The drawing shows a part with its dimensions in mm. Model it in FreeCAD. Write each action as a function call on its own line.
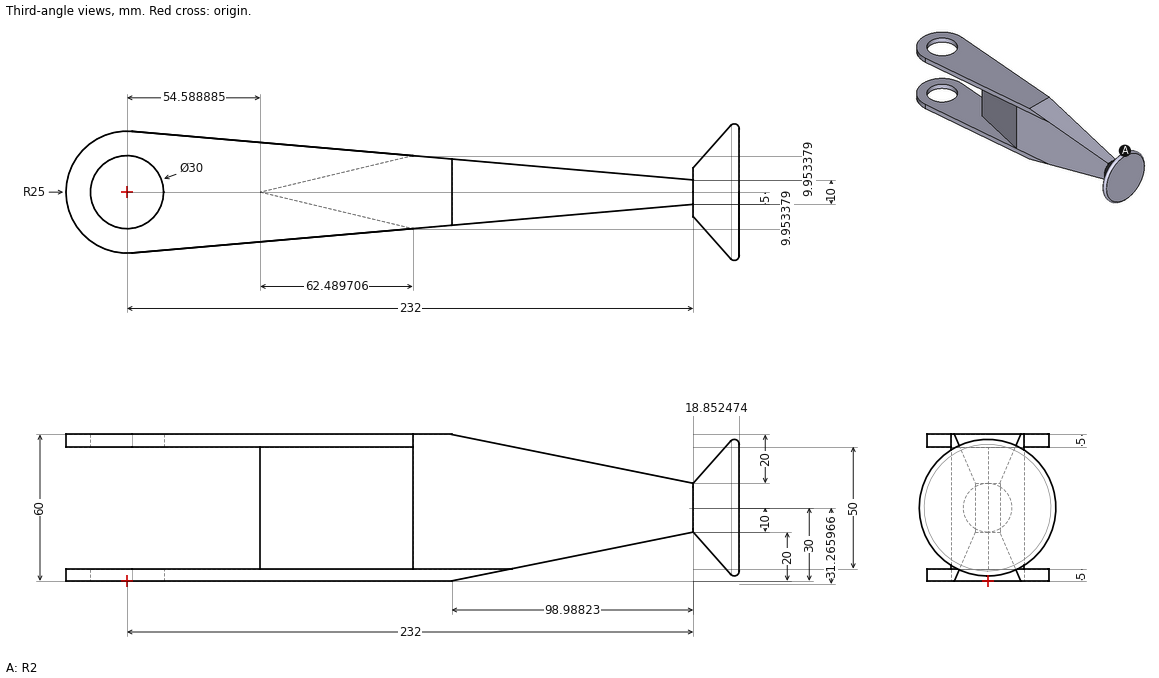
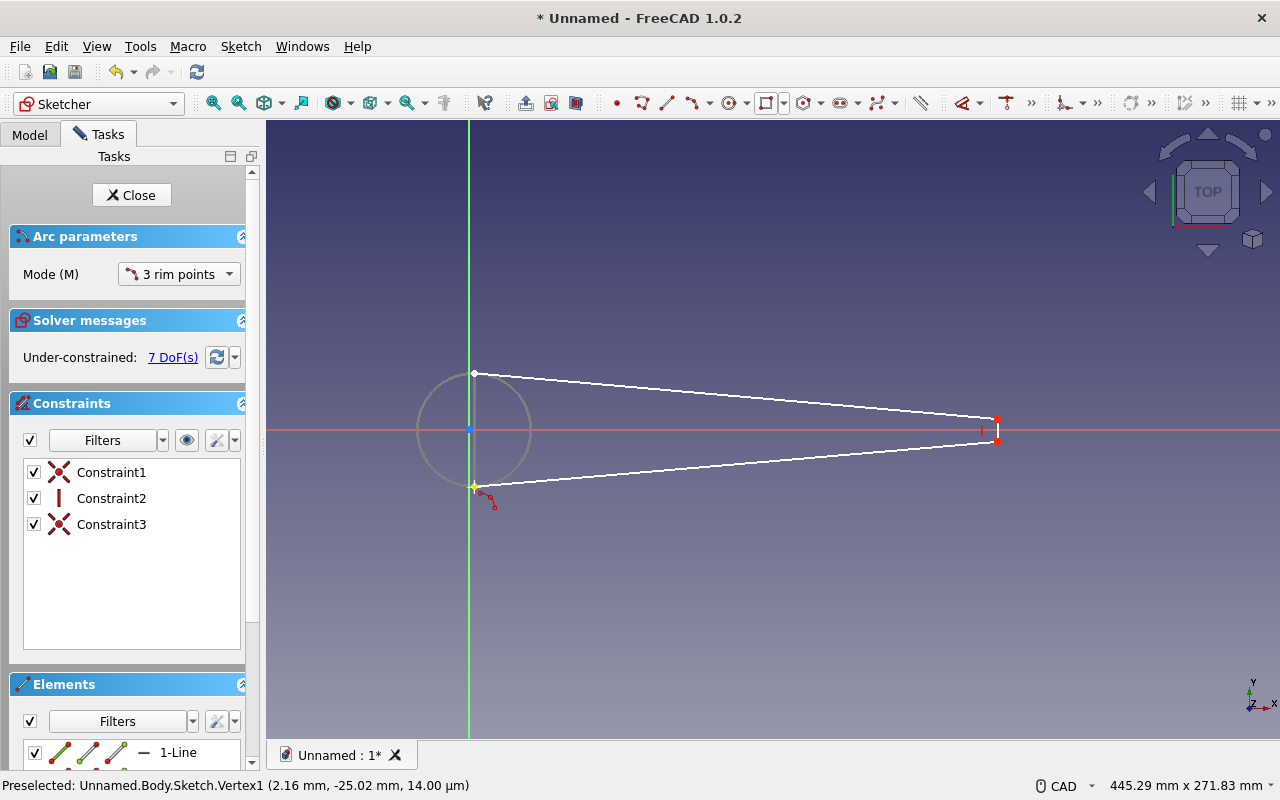
click(415, 411)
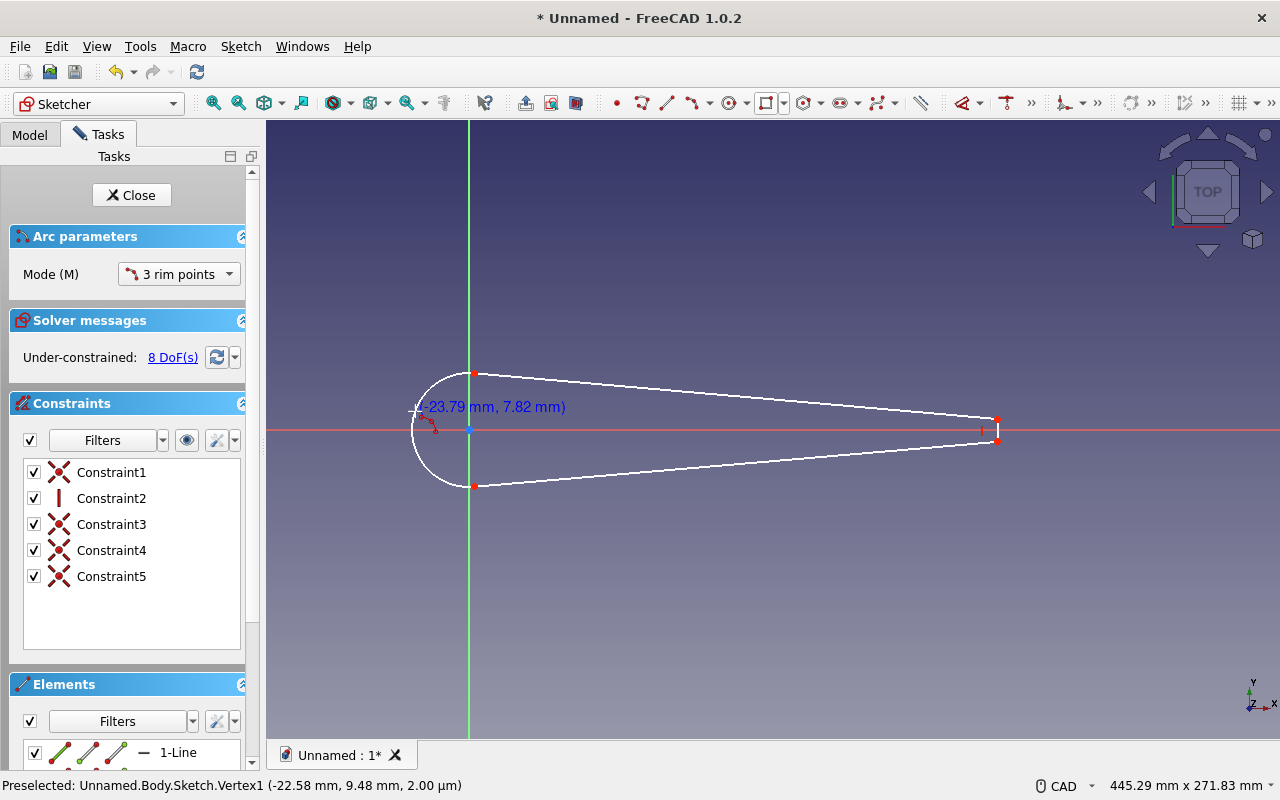
click(728, 104)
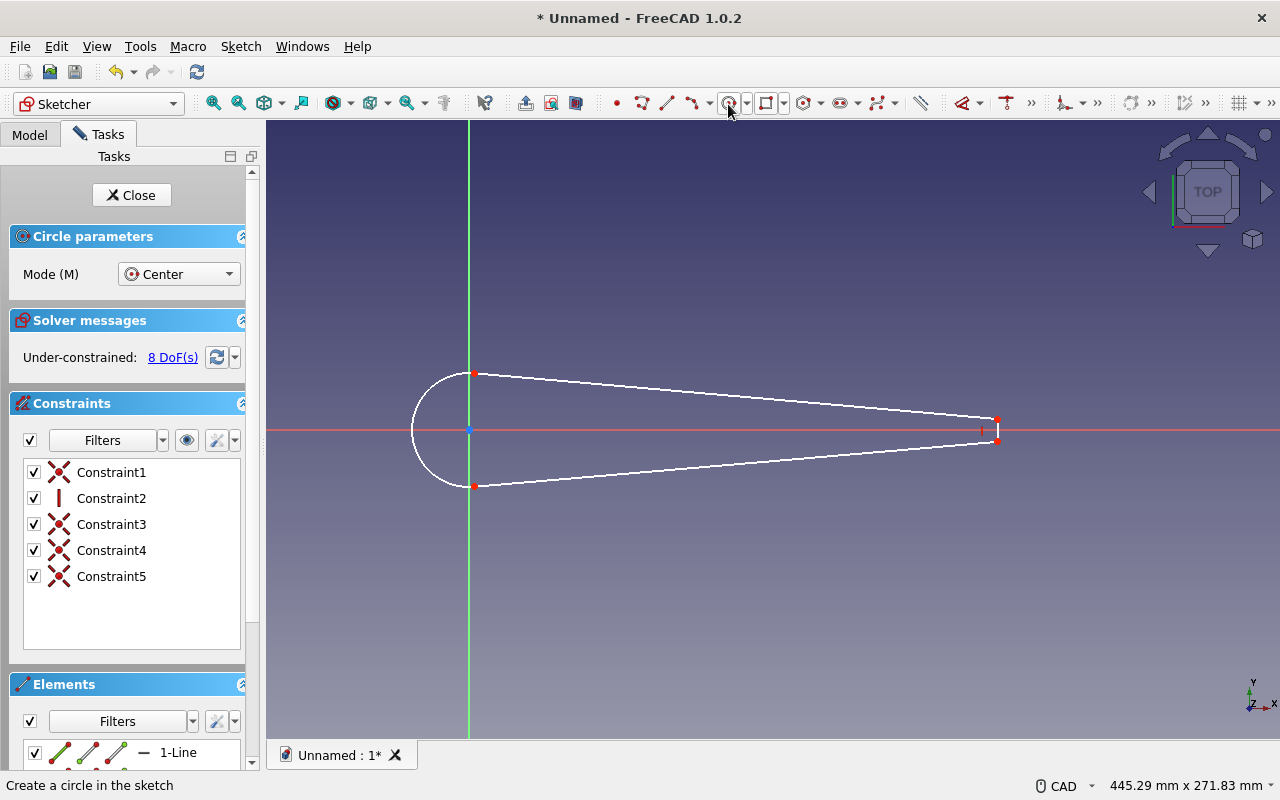
click(469, 430)
click(493, 406)
key(Escape)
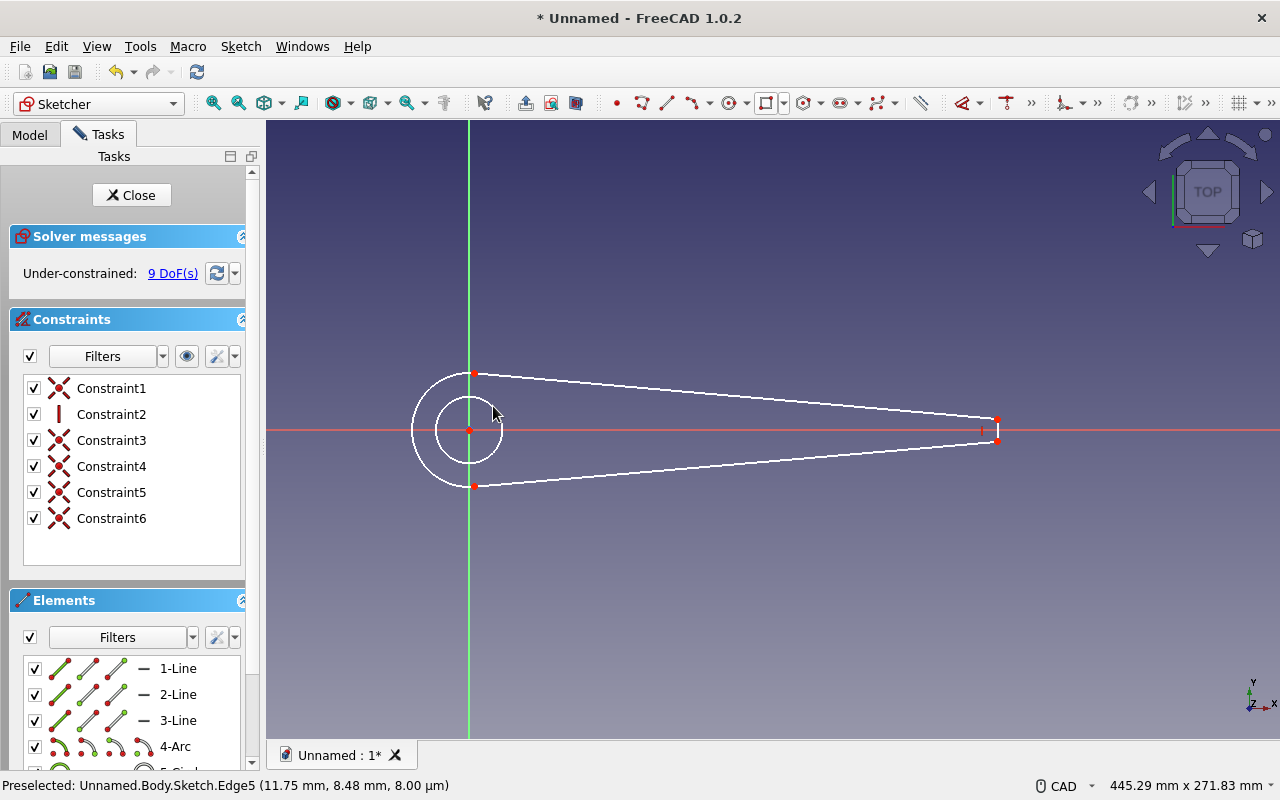
click(631, 473)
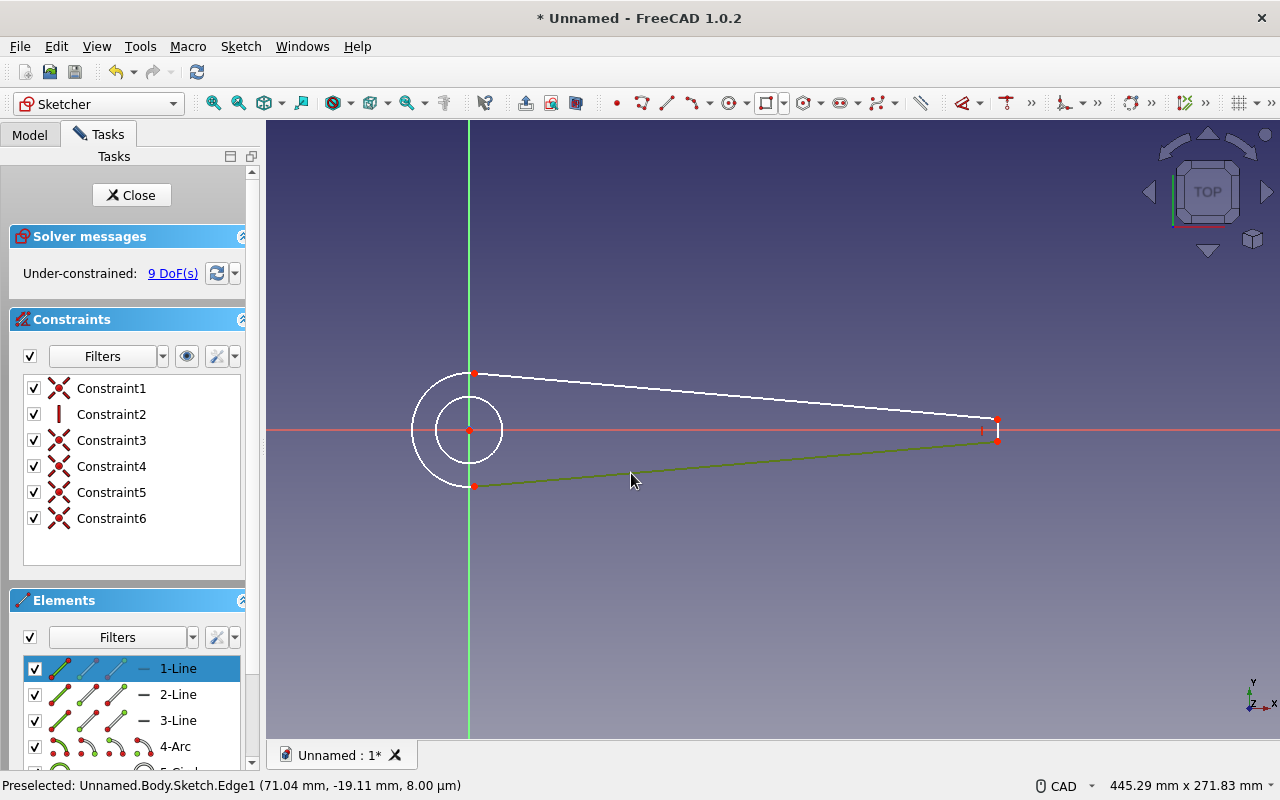
click(424, 395)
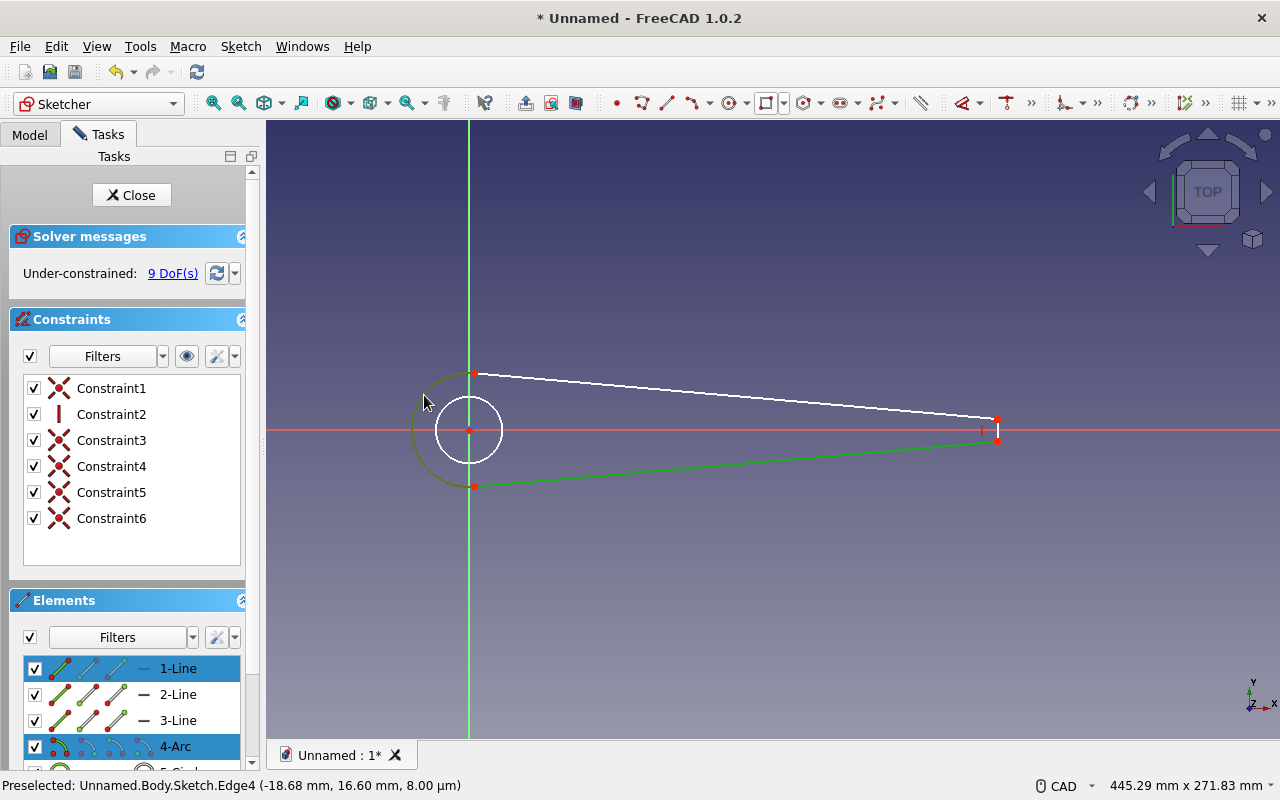
key(t)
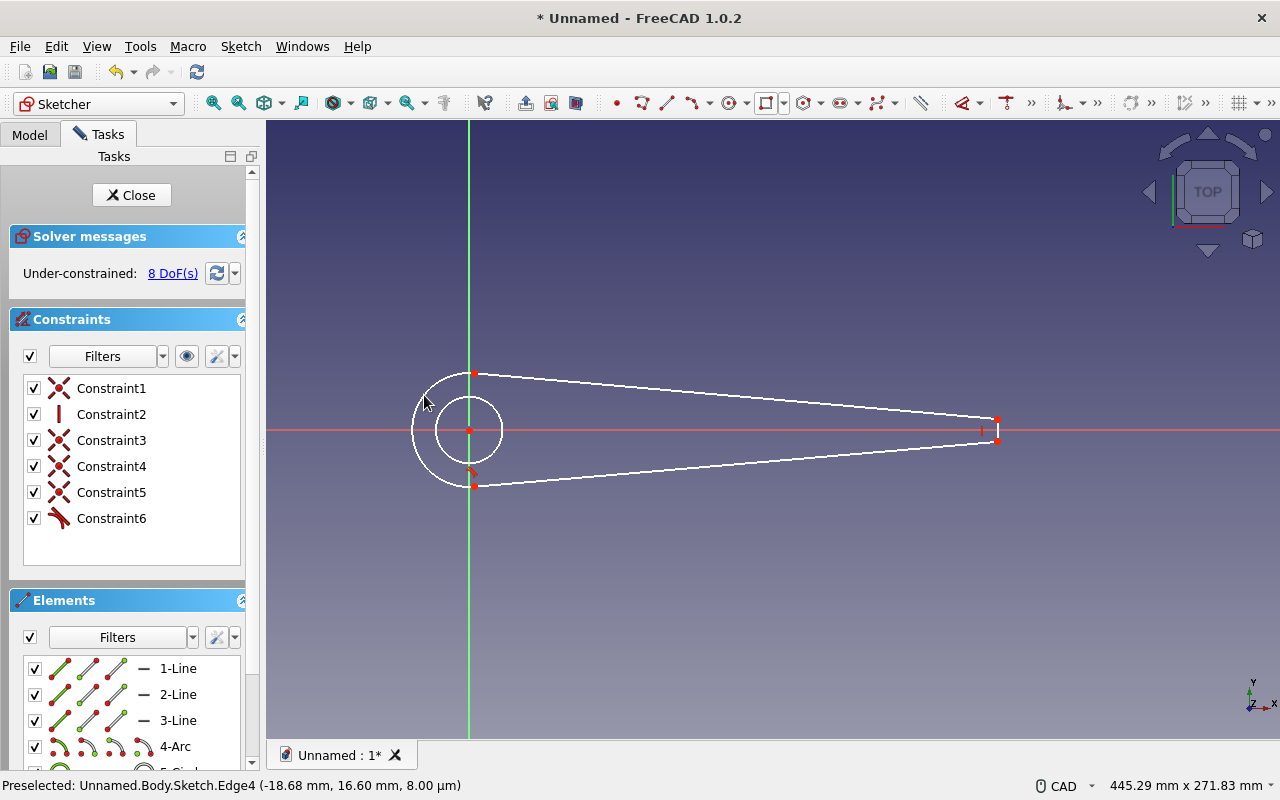
click(841, 405)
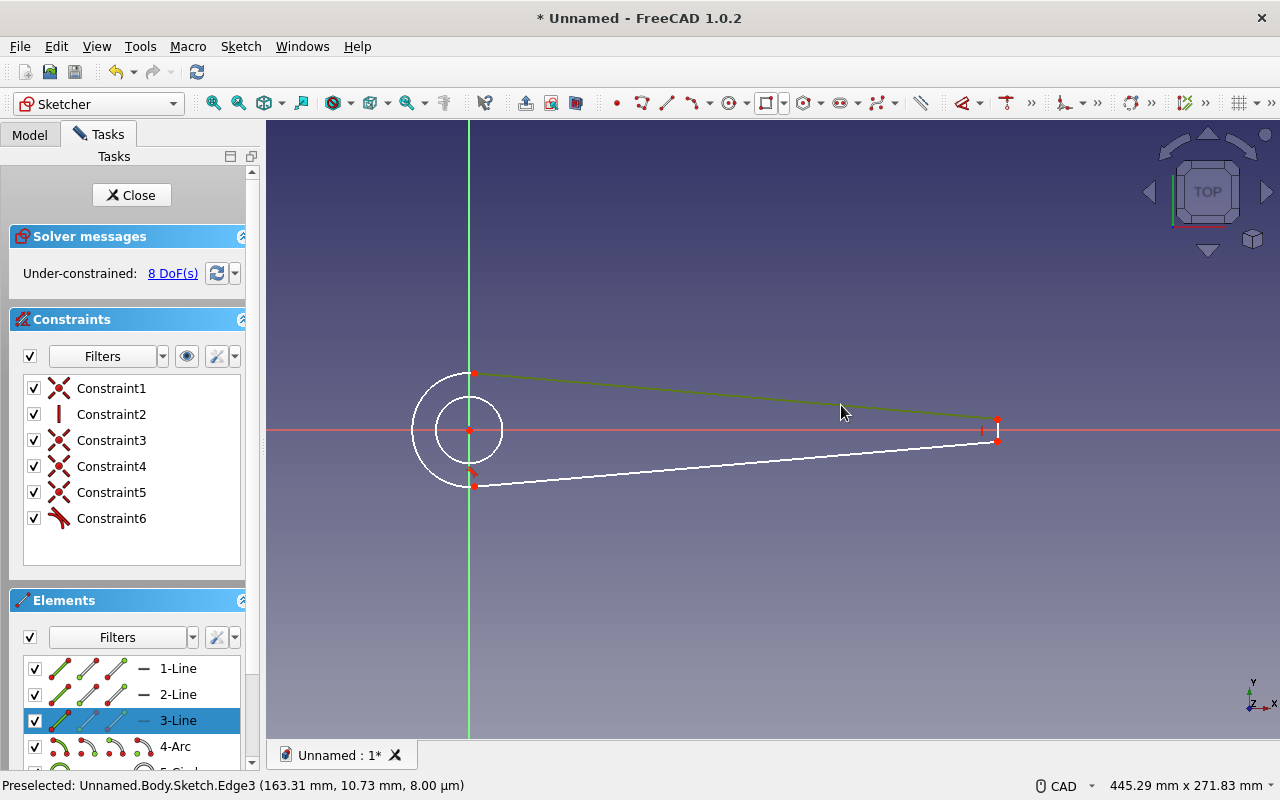
click(424, 395)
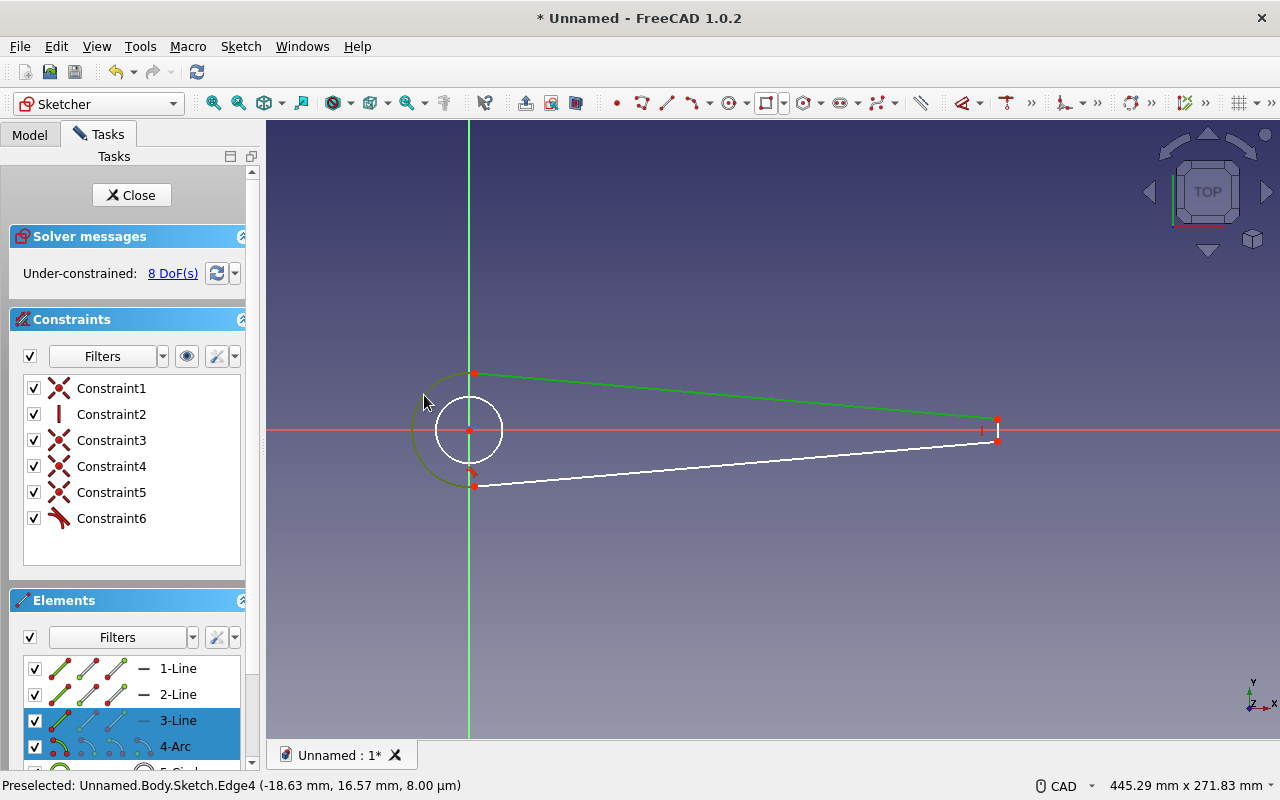
key(t)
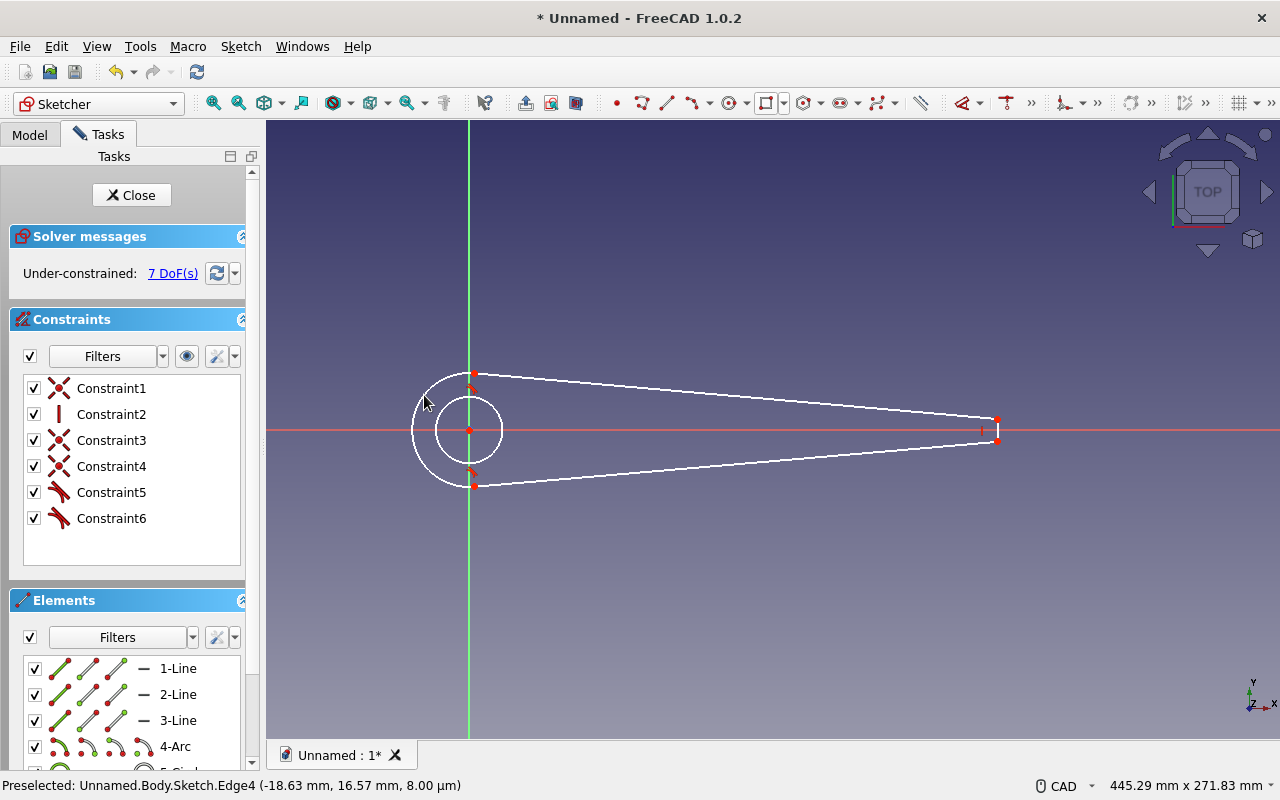
drag(459, 420, 479, 440)